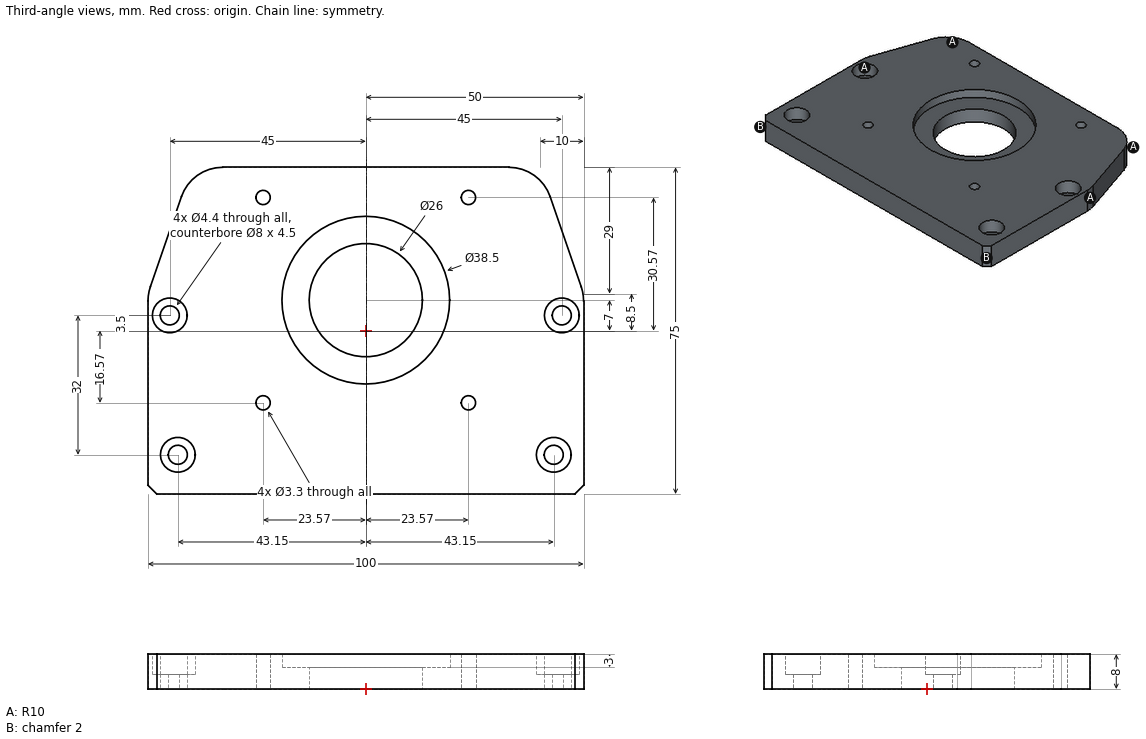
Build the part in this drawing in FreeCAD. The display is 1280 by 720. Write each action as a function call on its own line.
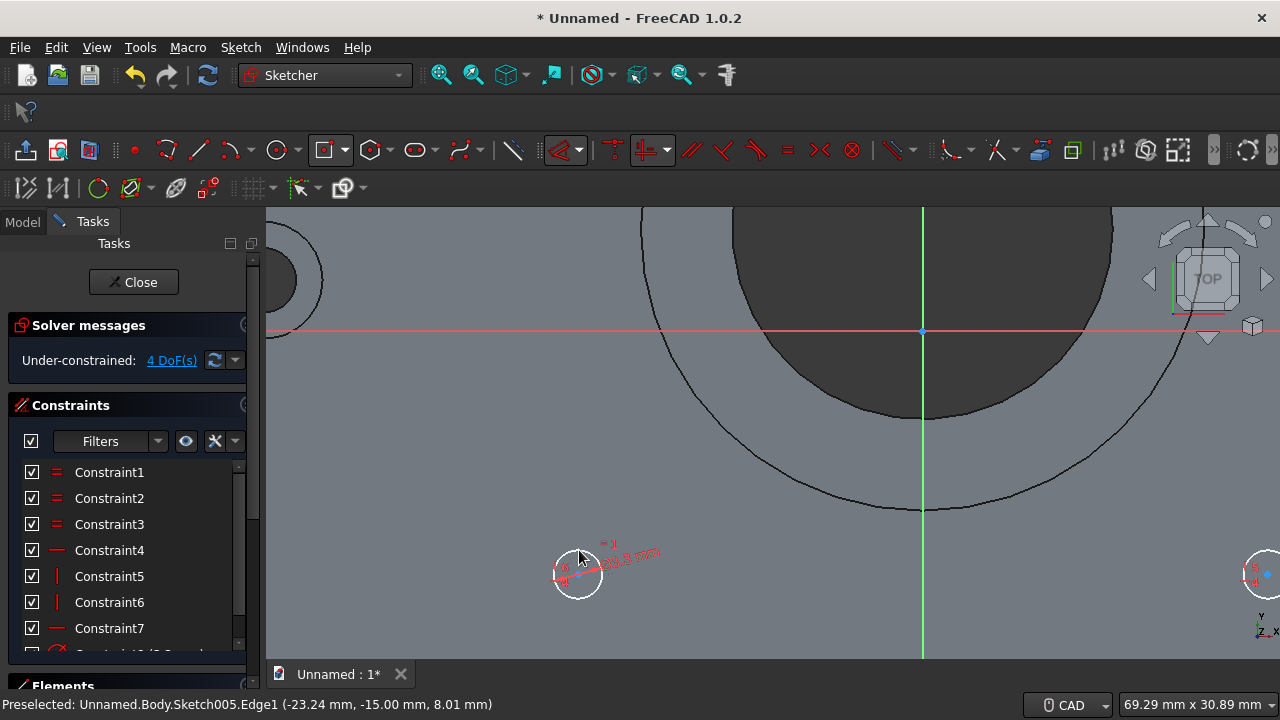
click(578, 574)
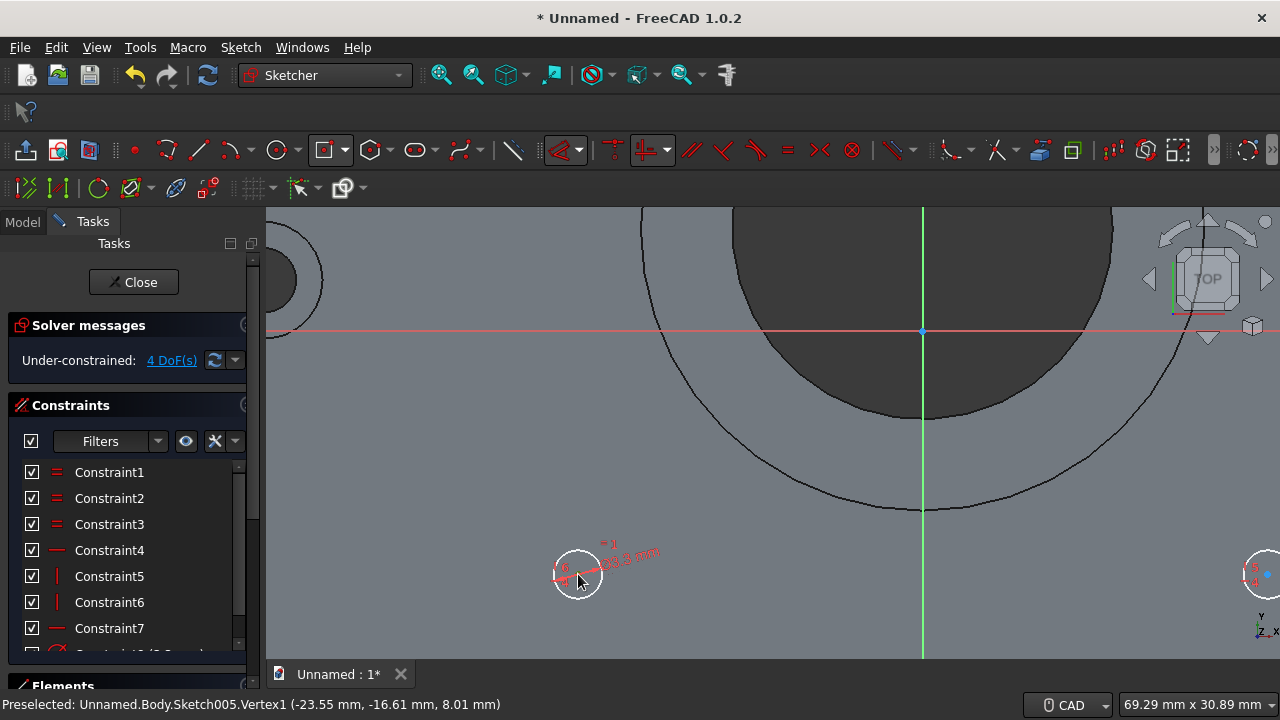
key(l)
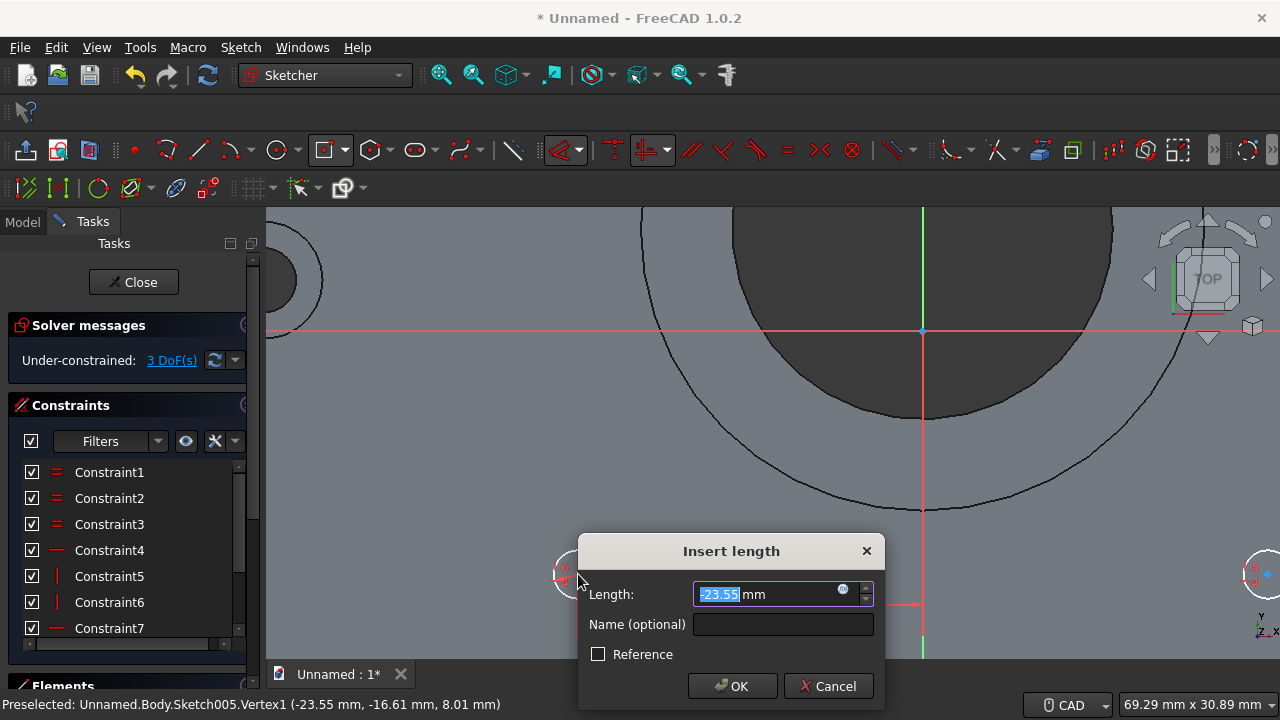
text(-23.57)
key(Return)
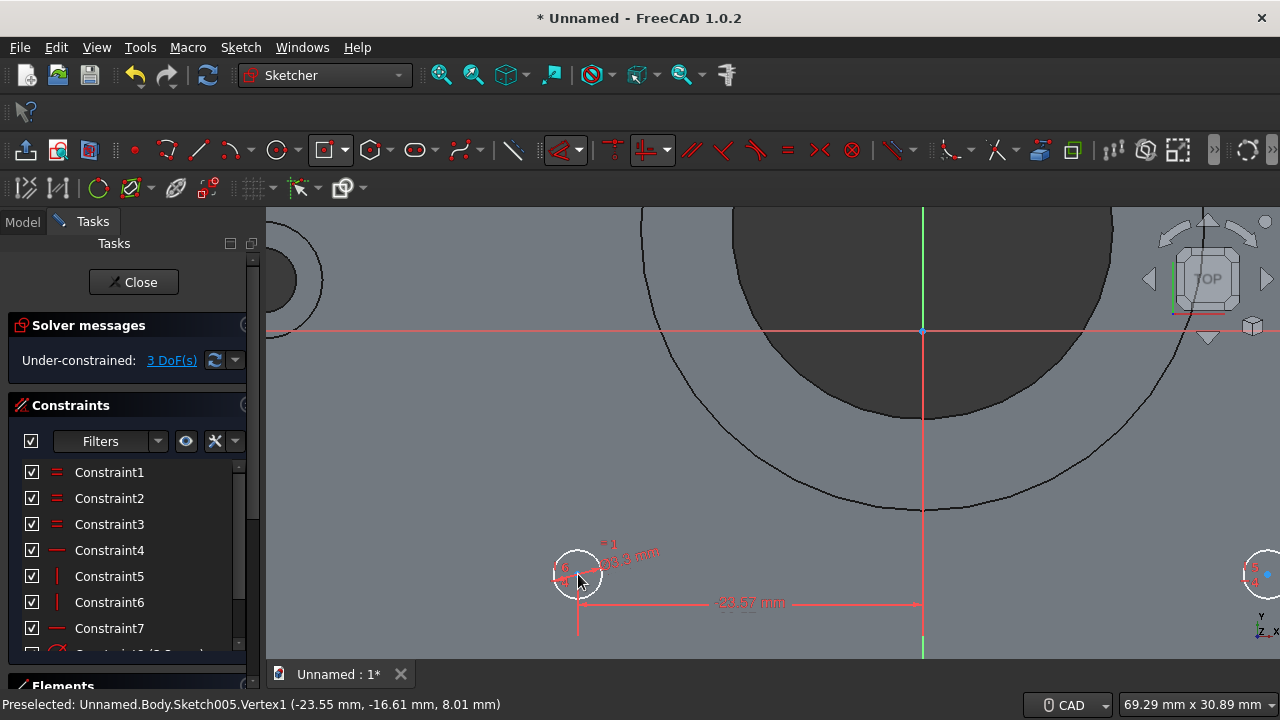
click(578, 574)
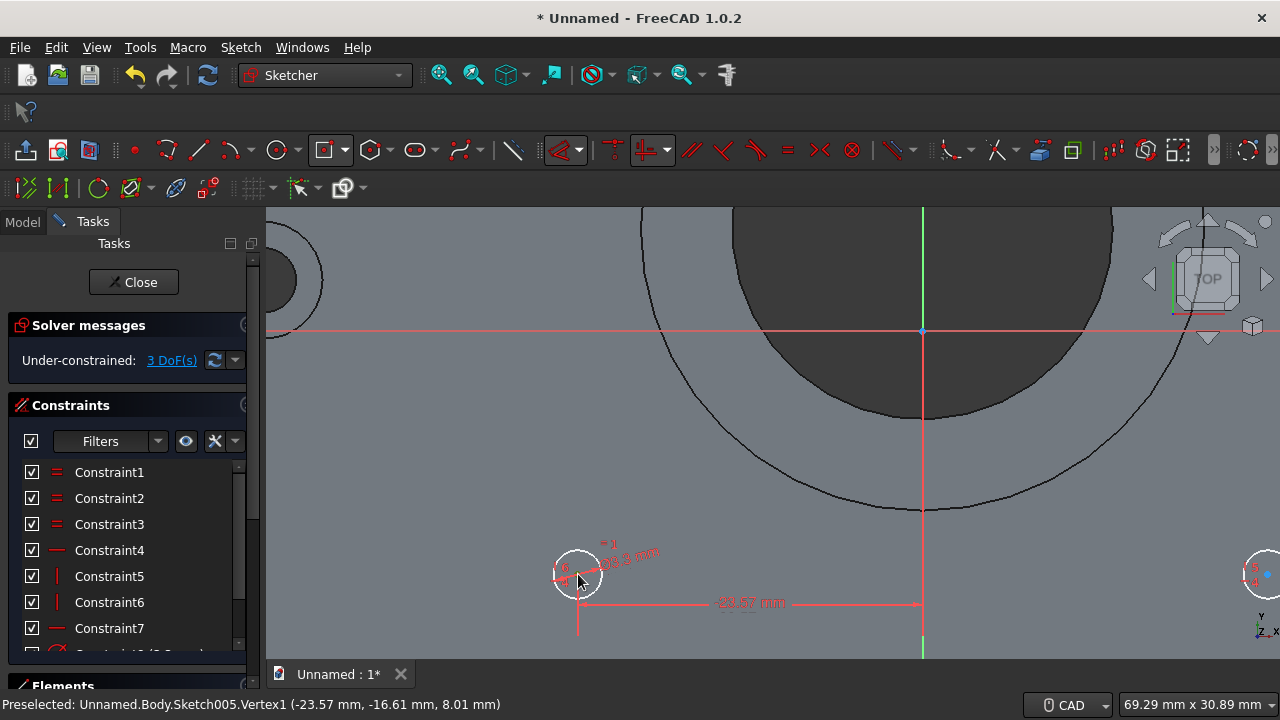
key(i)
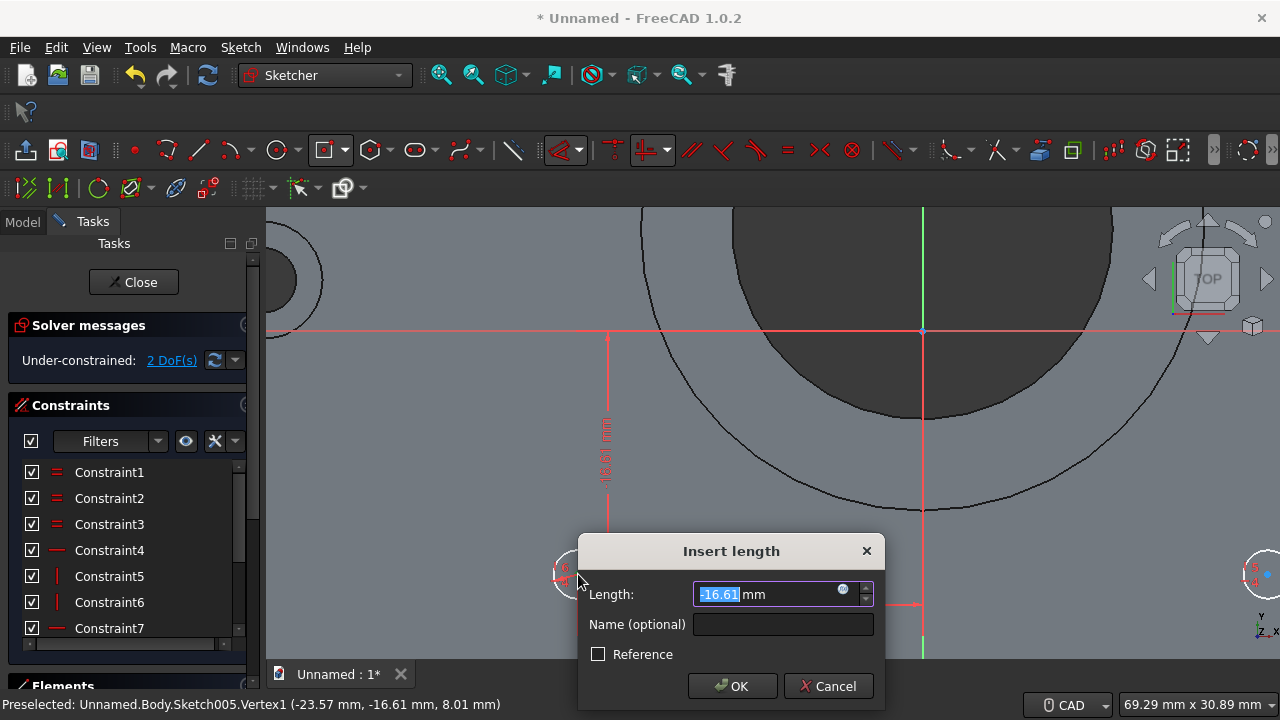
text(-16.57)
key(Return)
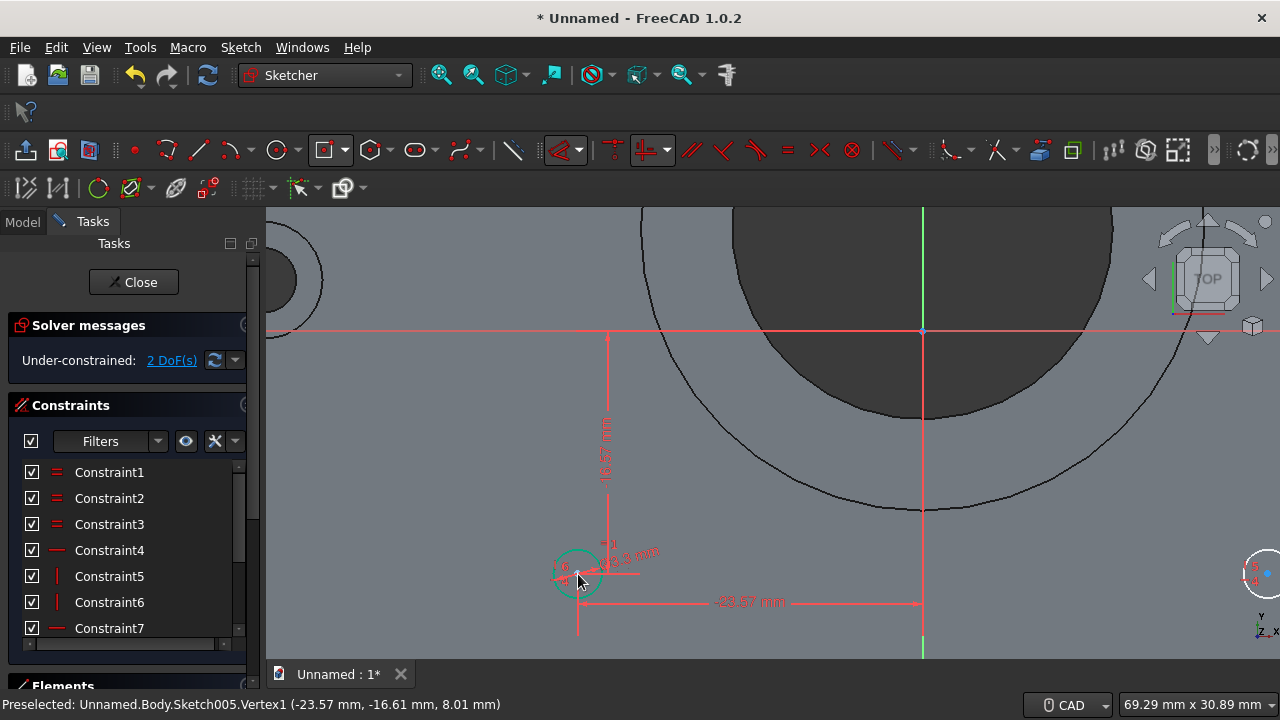
scroll(578, 552, down, 5)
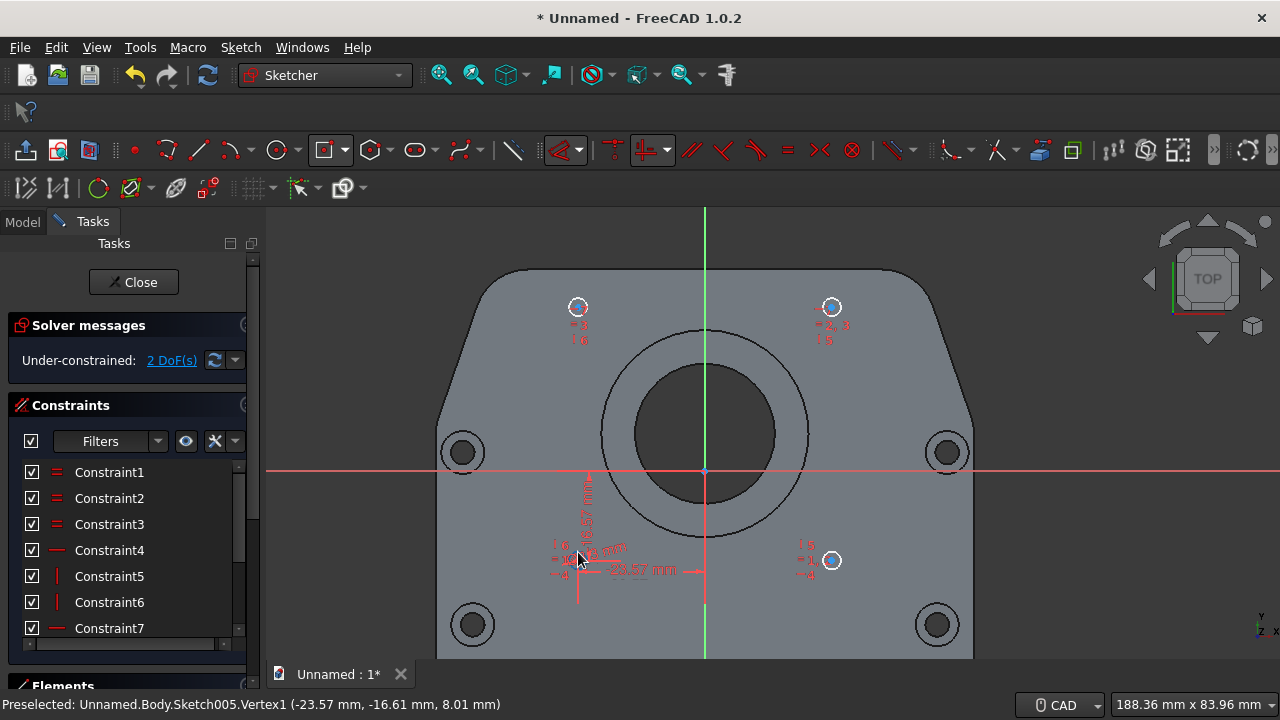
click(832, 561)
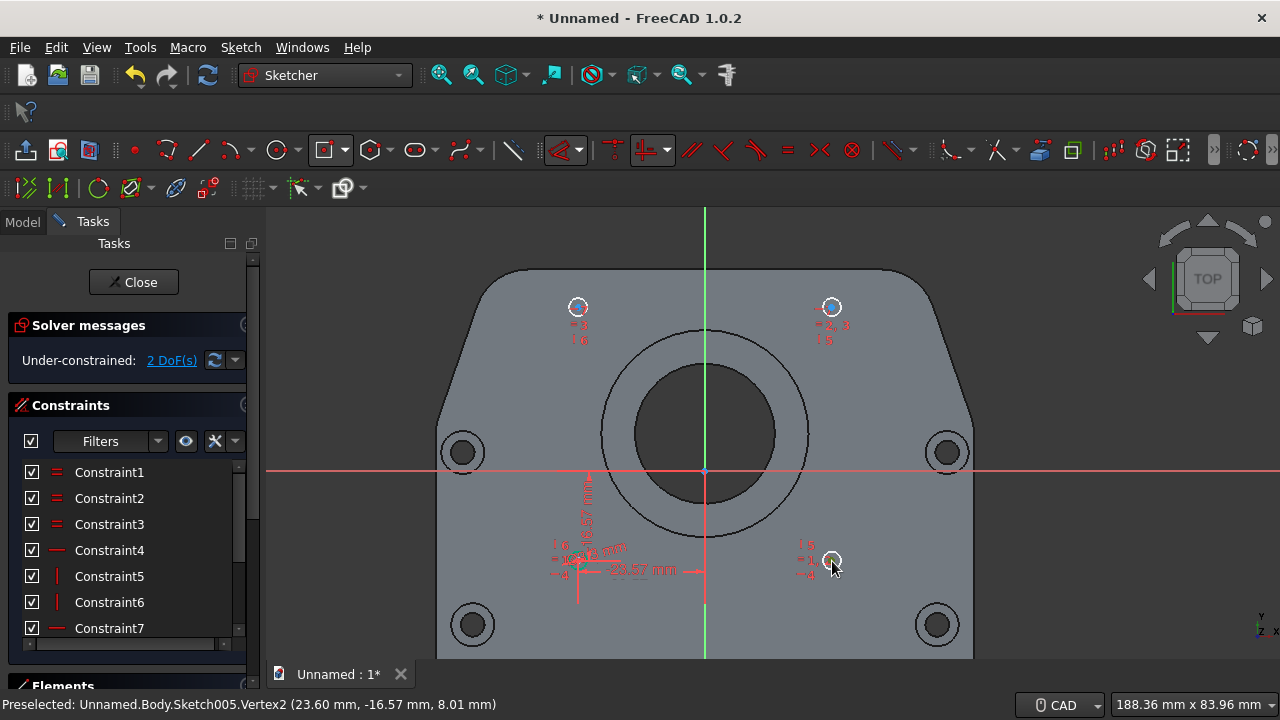
click(582, 150)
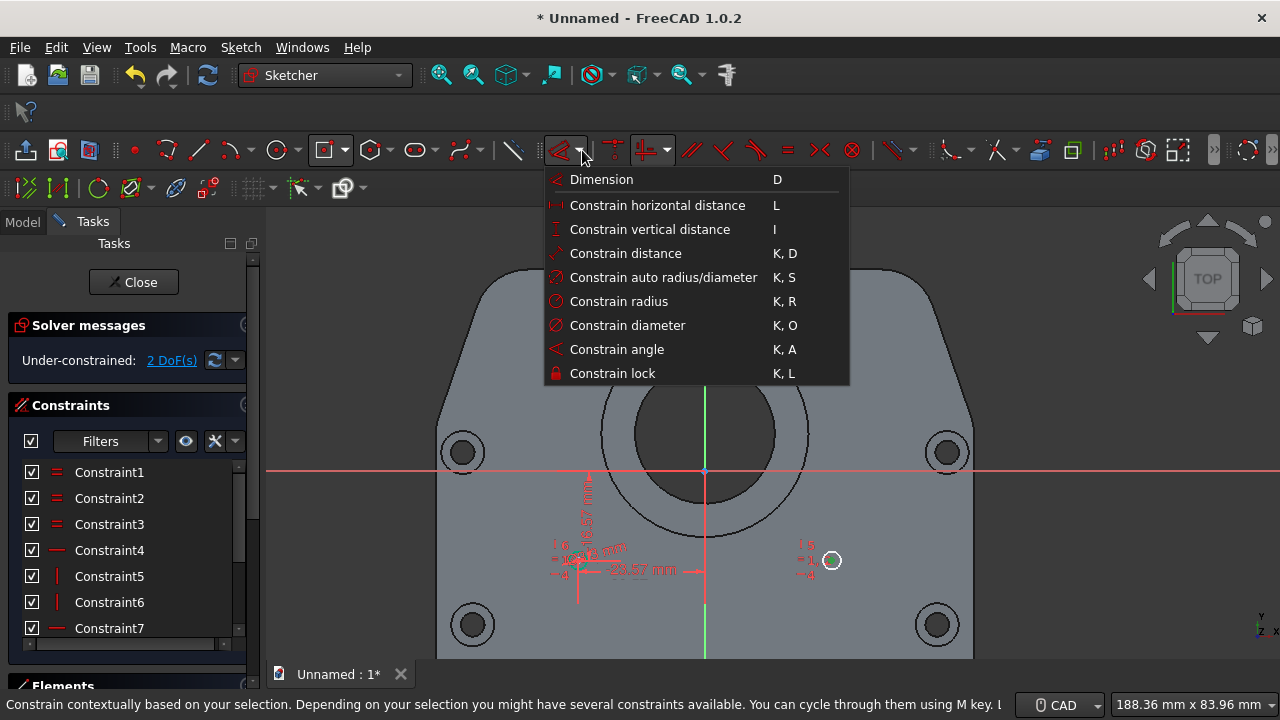
click(697, 205)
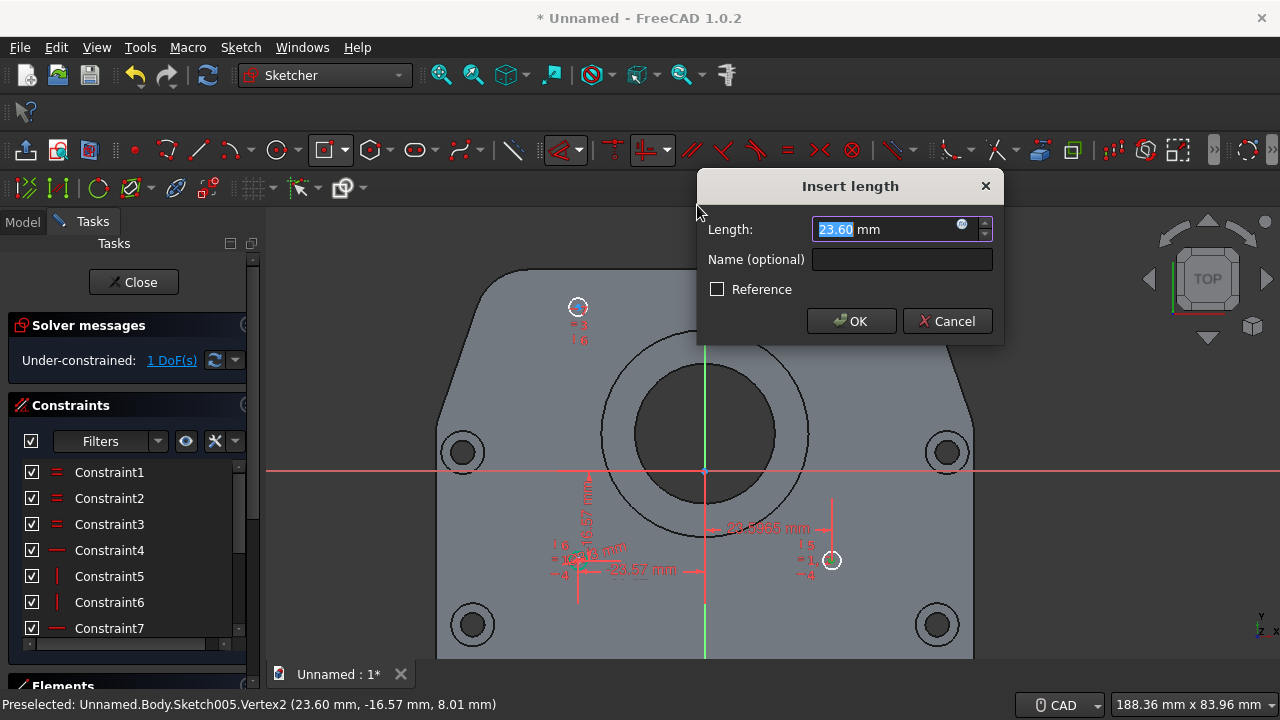
text(23.57)
key(Return)